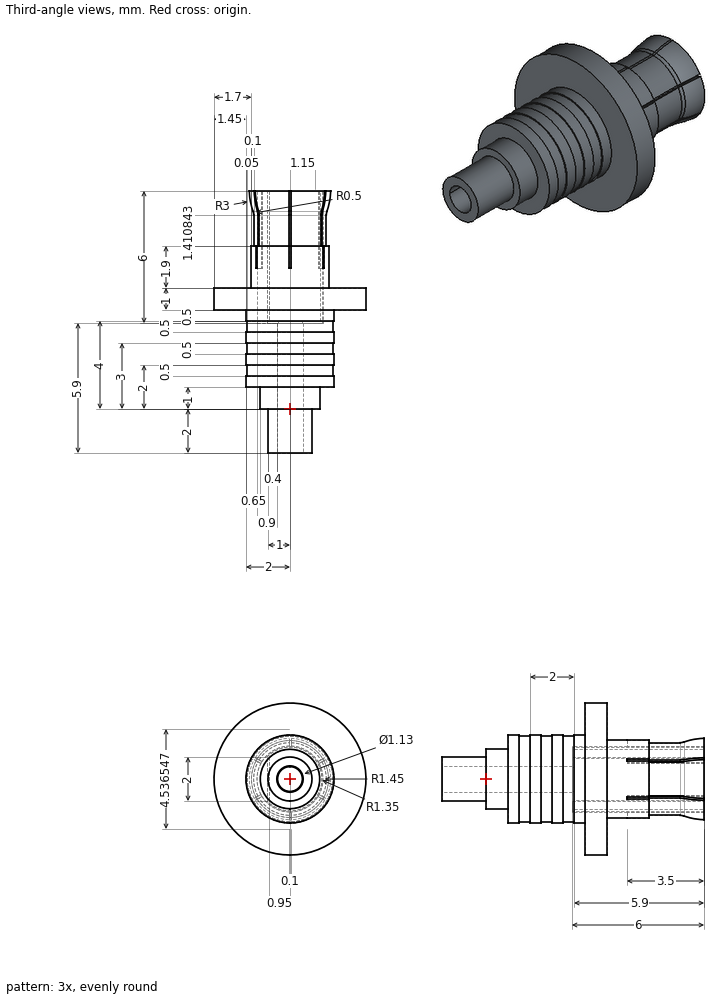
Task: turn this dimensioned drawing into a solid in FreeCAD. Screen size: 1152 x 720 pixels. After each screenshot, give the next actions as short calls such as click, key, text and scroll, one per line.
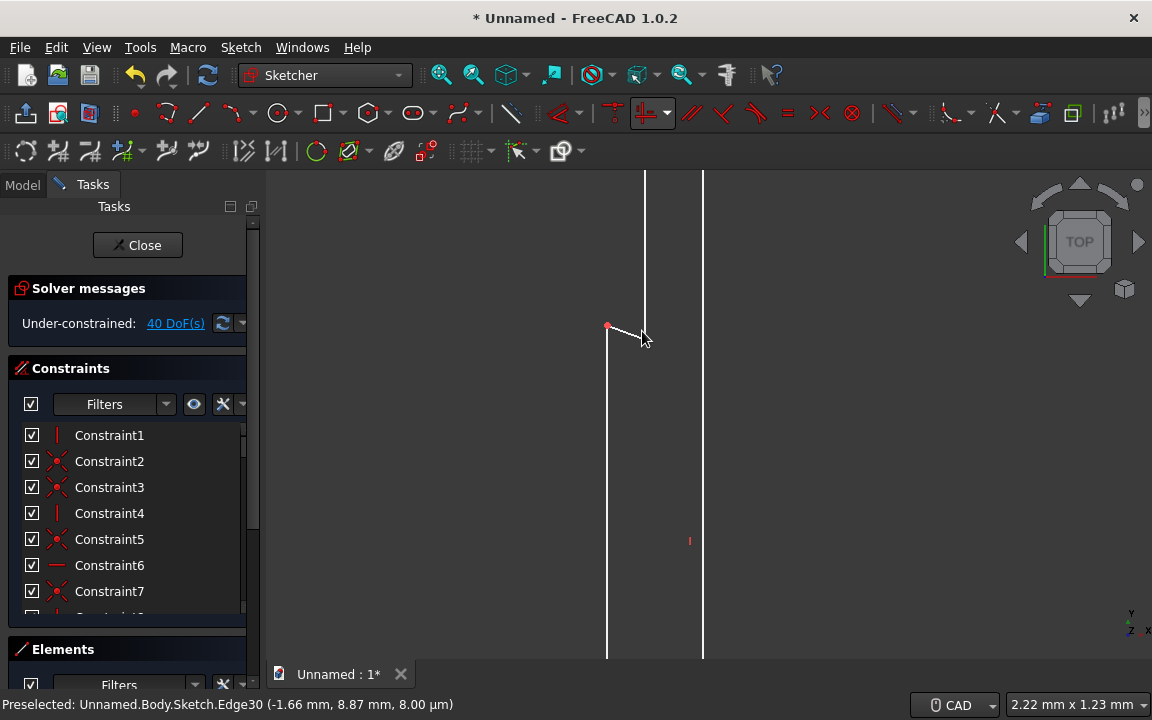
click(630, 334)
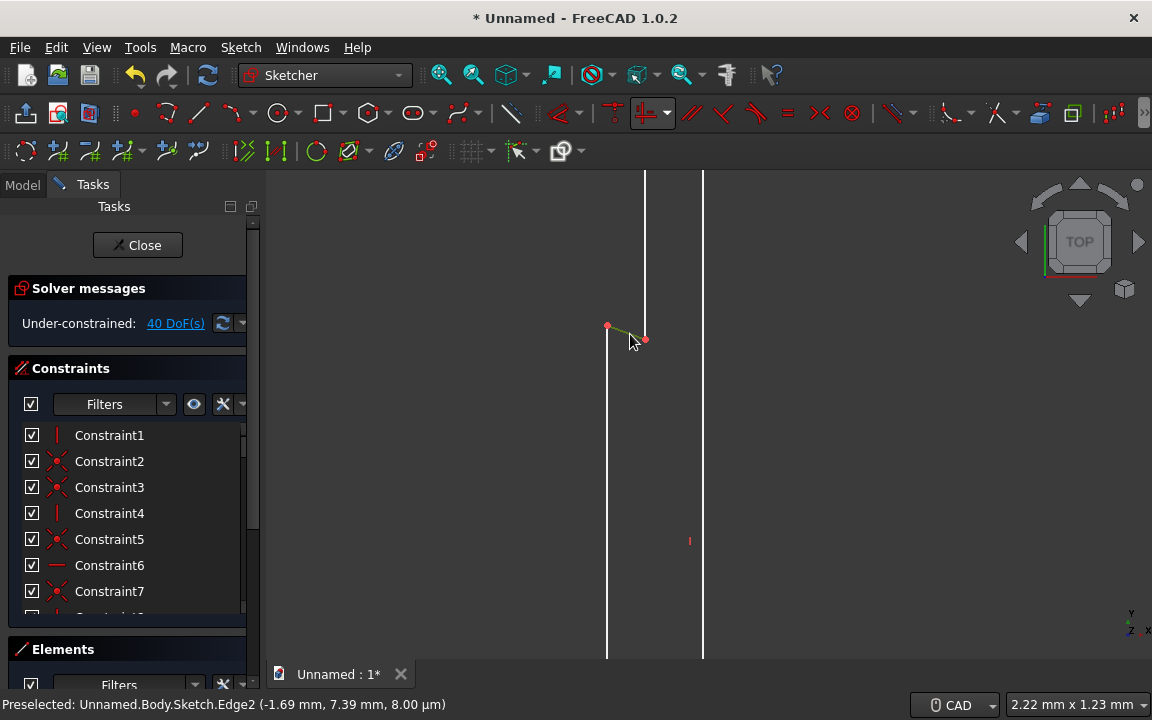
key(h)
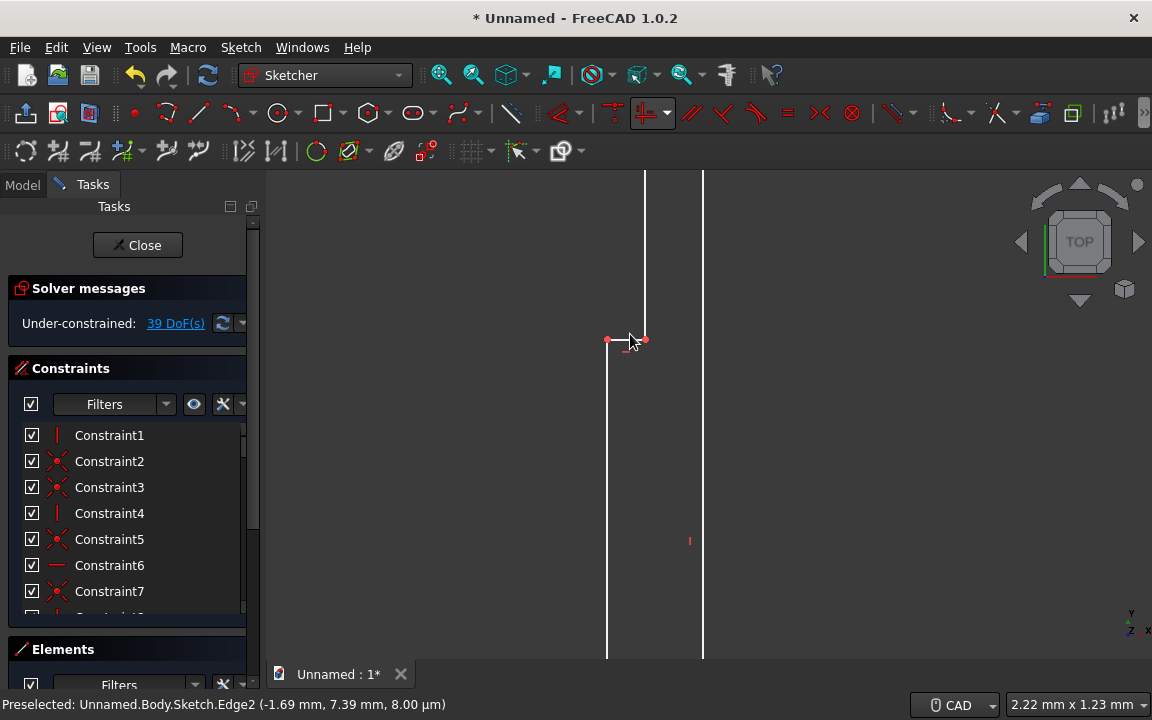
scroll(642, 331, down, 14)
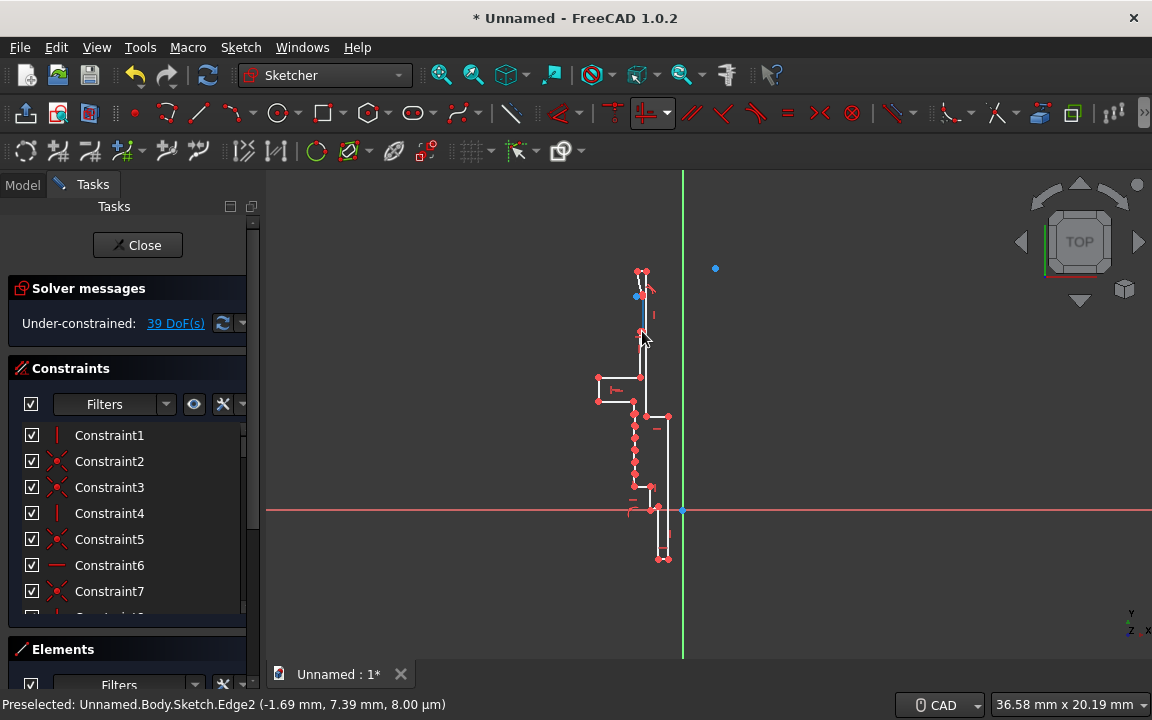
scroll(634, 414, up, 14)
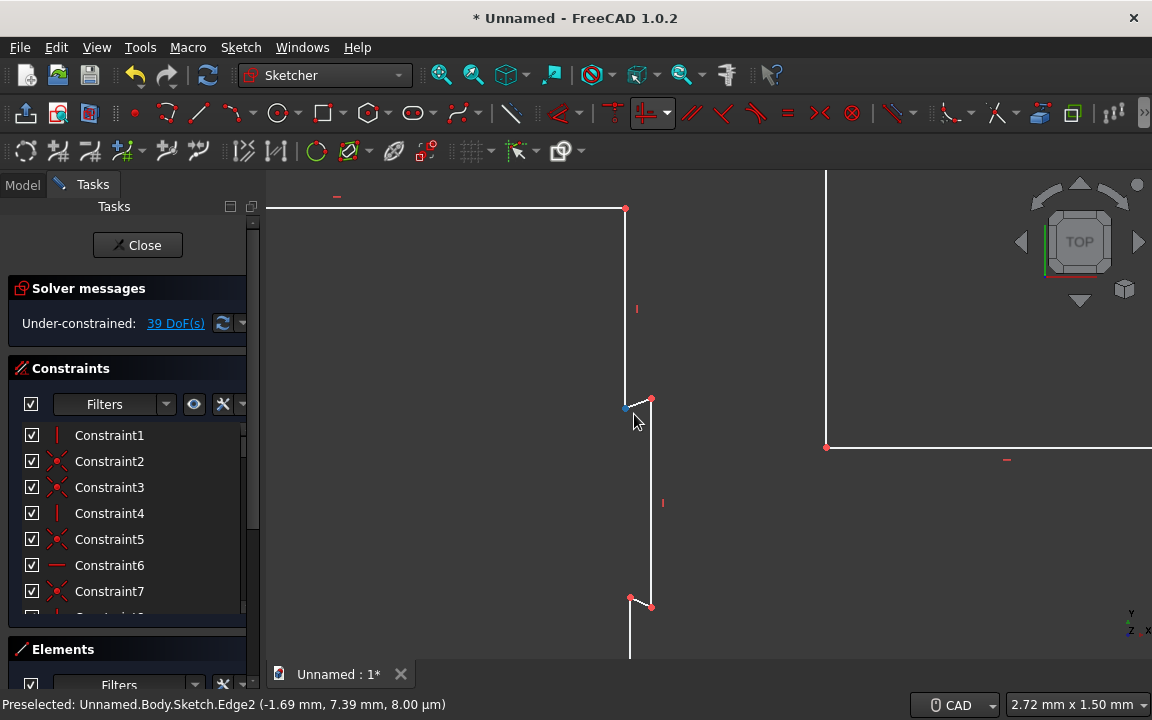
click(636, 405)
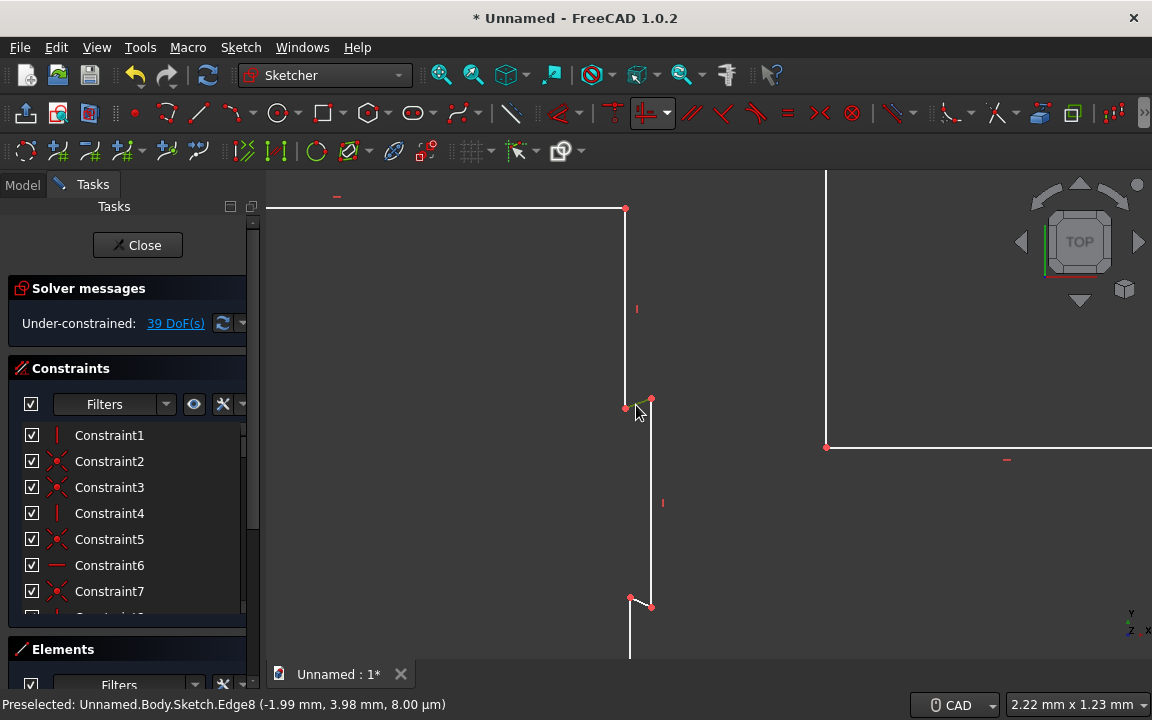
click(670, 114)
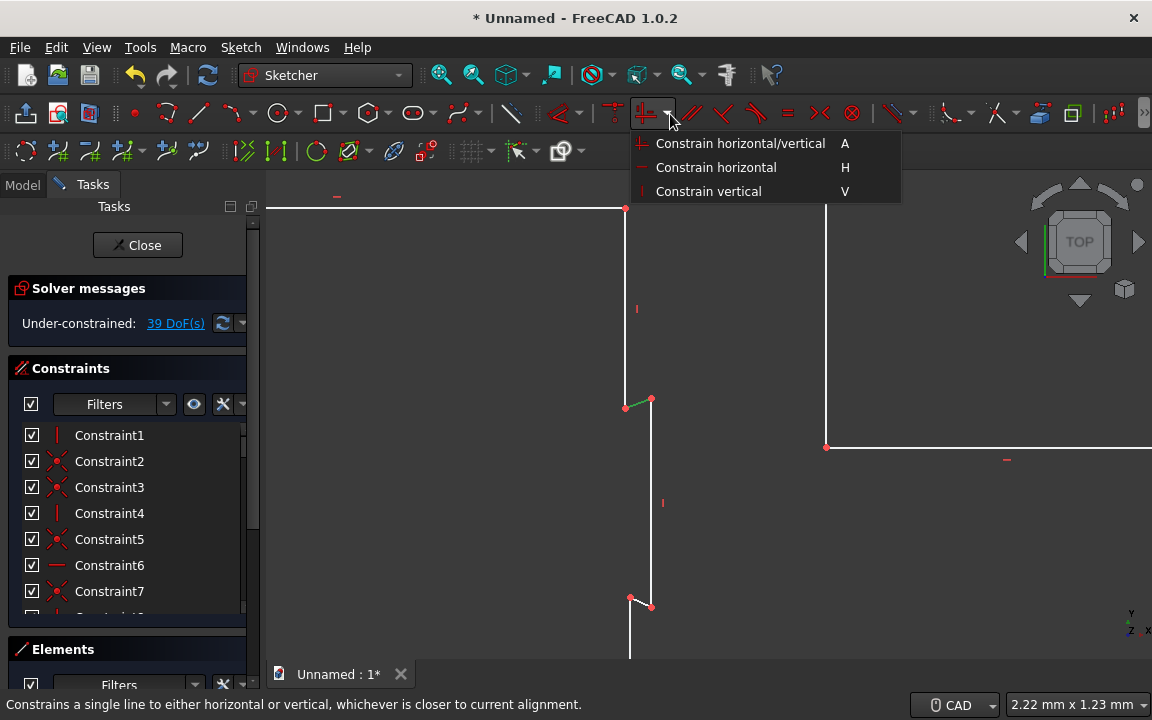
click(766, 167)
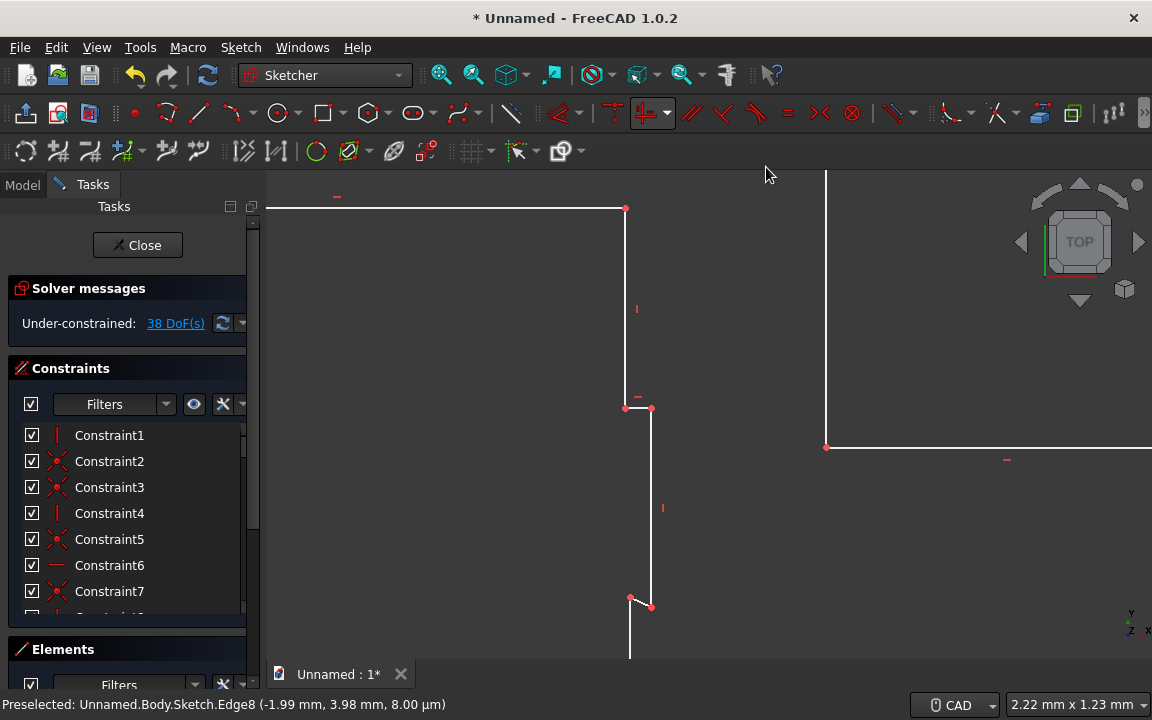
click(641, 602)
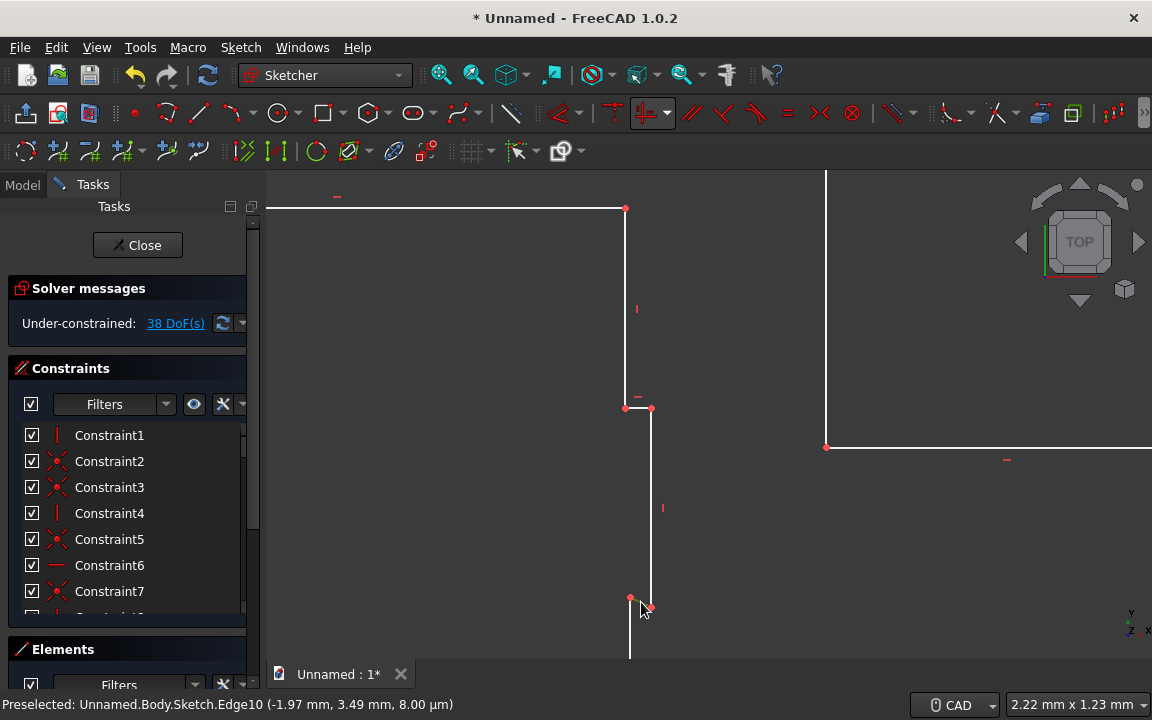
click(670, 114)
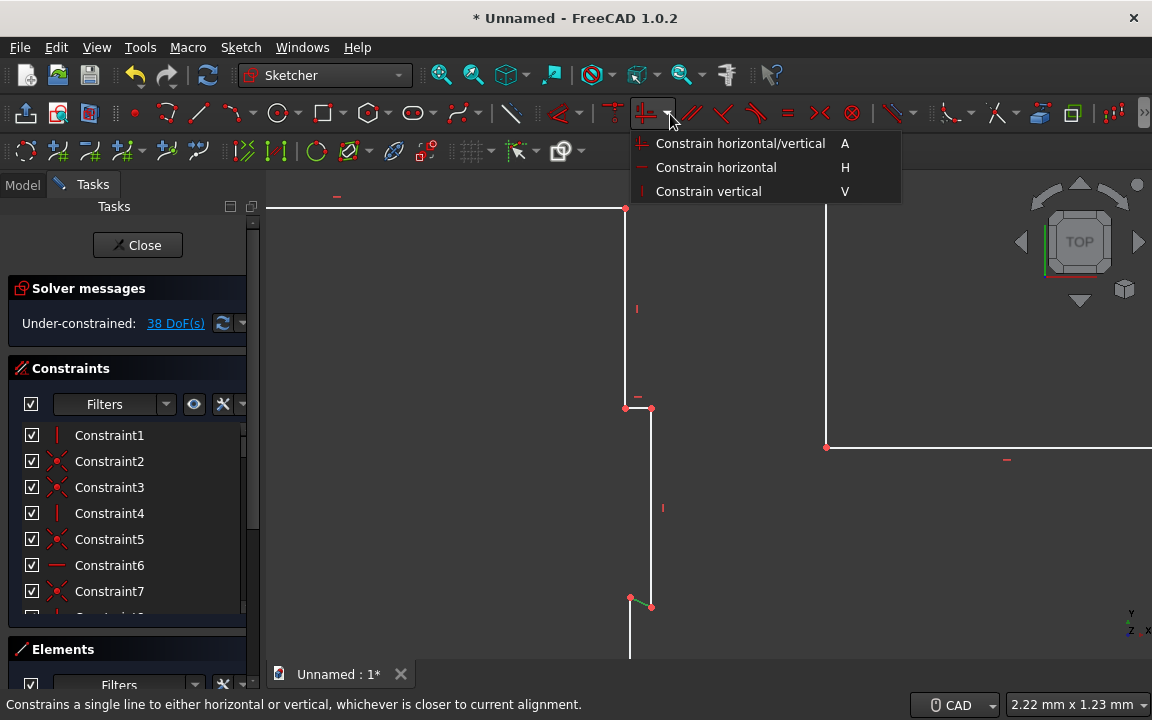
click(766, 167)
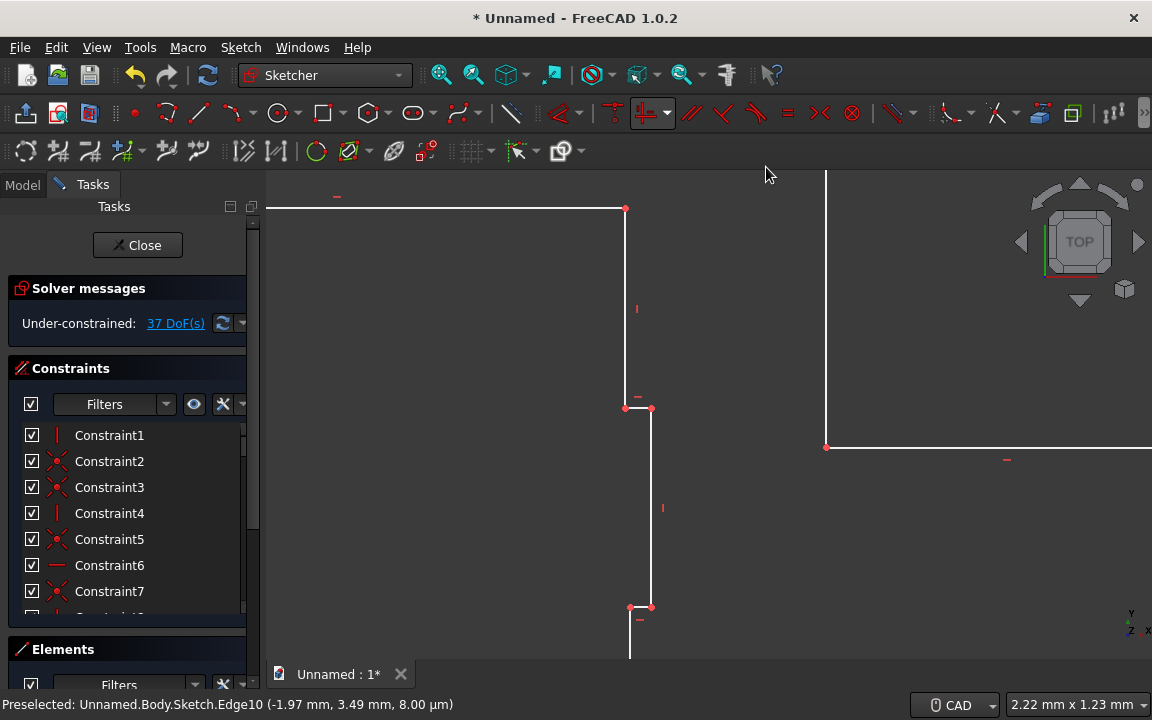
scroll(634, 414, down, 14)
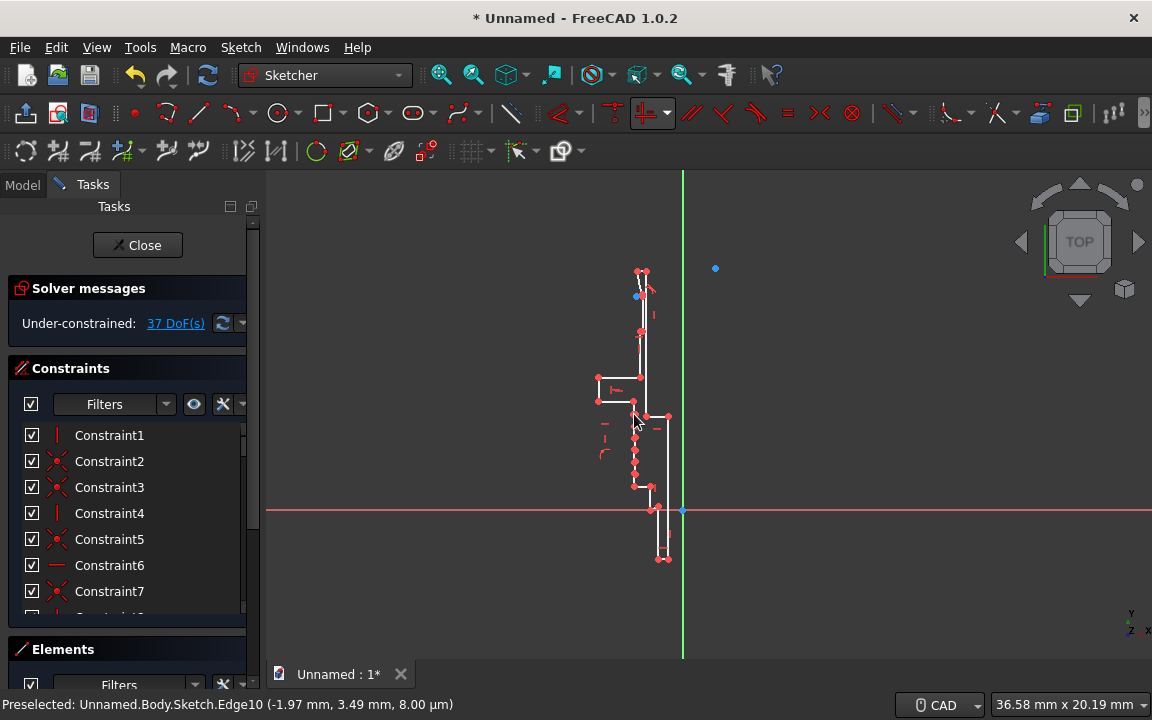
scroll(635, 438, up, 14)